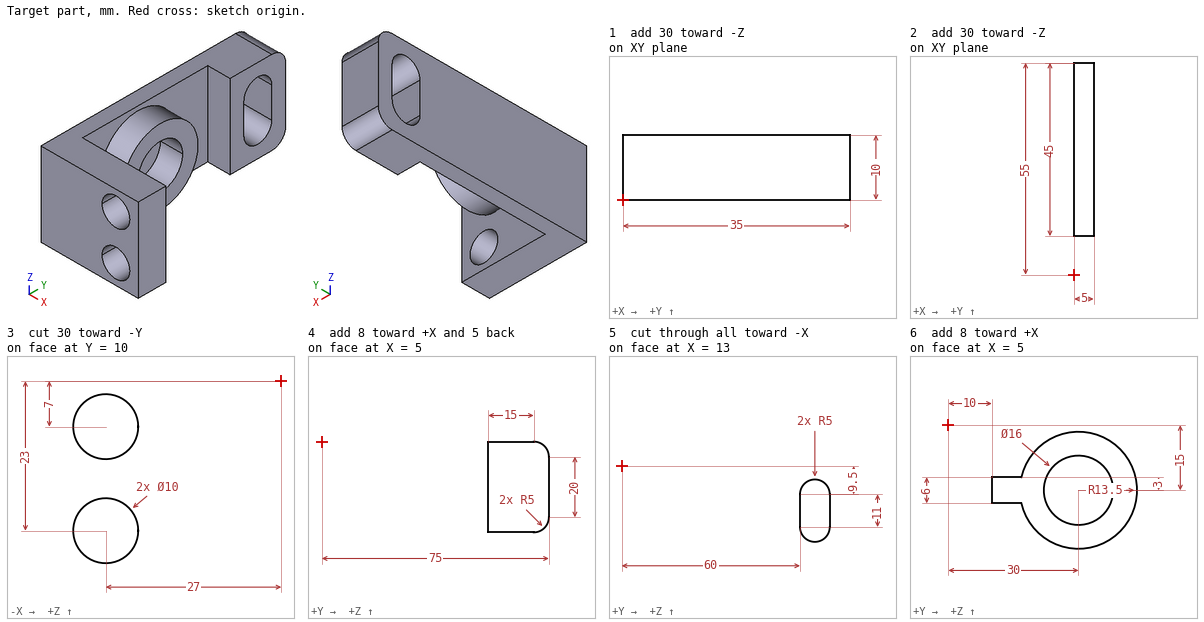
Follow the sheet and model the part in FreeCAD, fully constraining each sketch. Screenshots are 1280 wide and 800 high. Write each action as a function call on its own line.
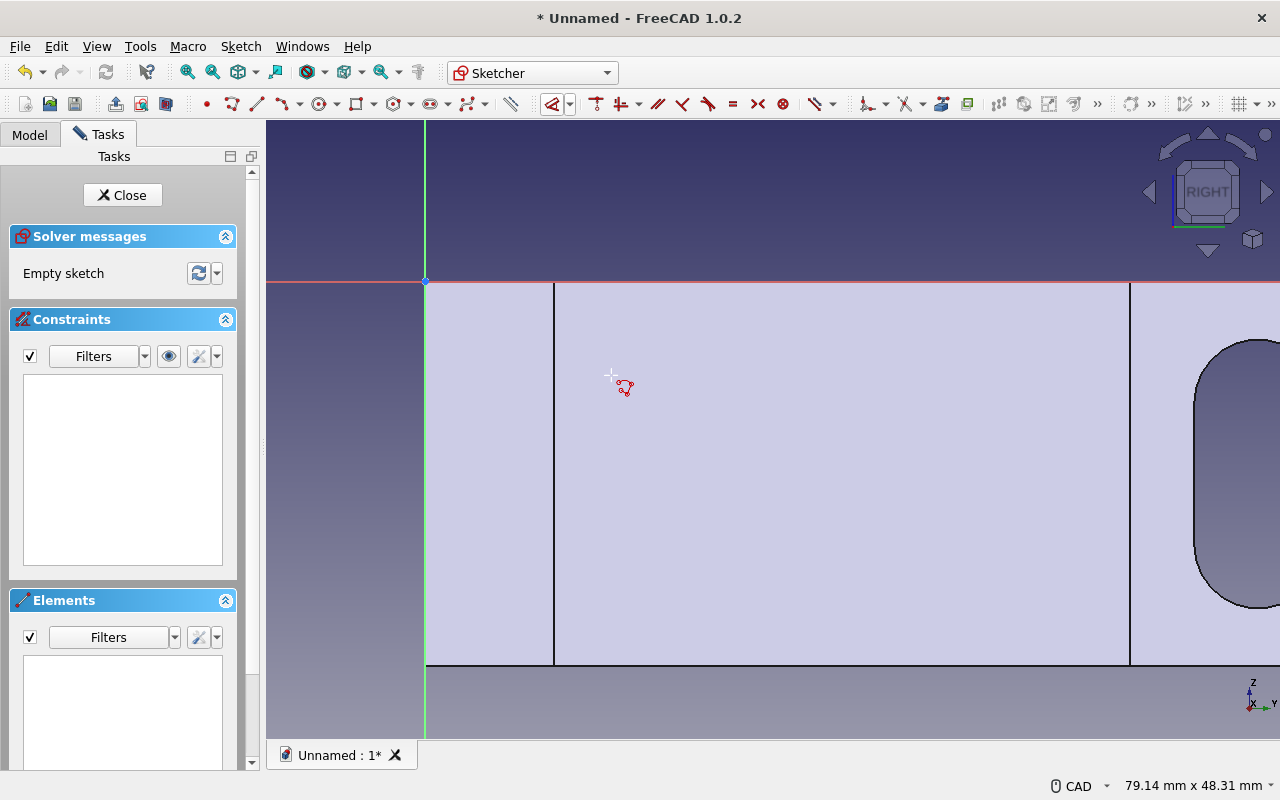
click(641, 436)
click(554, 436)
click(554, 512)
click(641, 512)
right_click(641, 512)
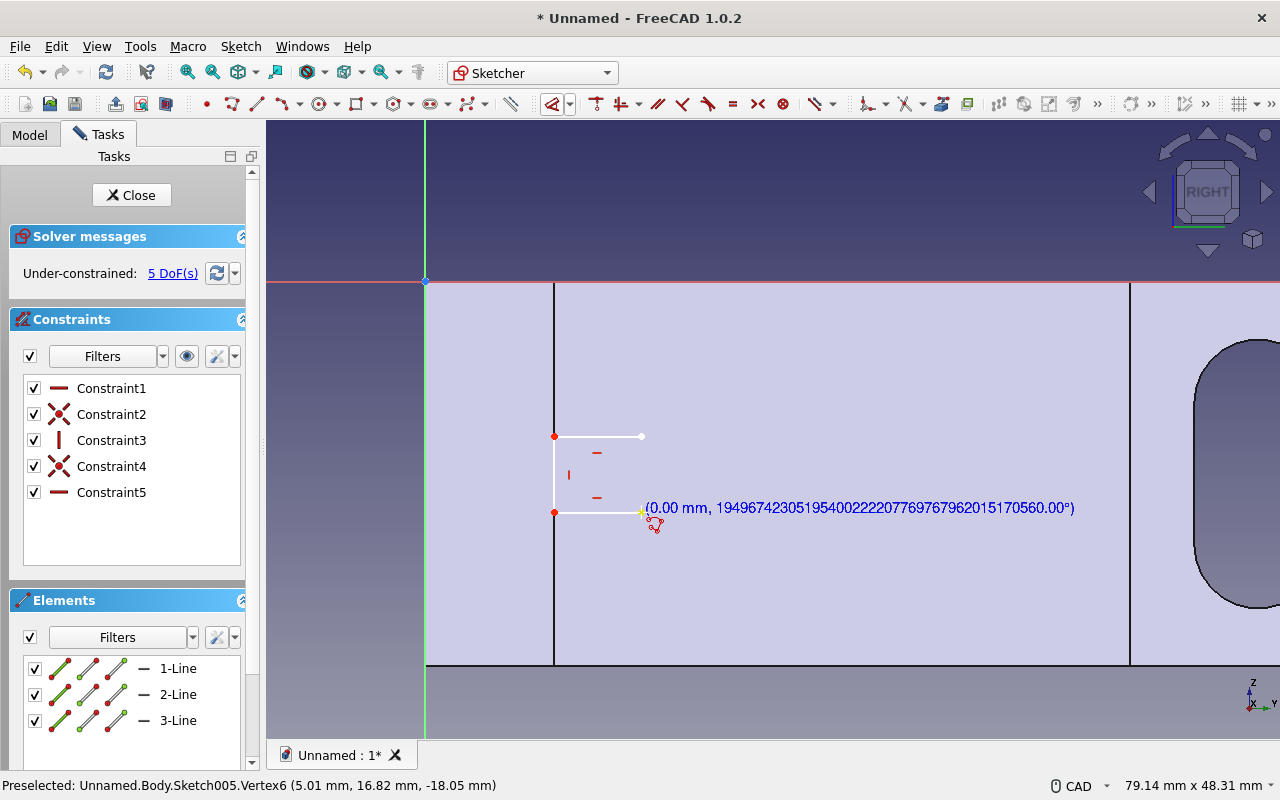
key(g)
key(3)
key(a)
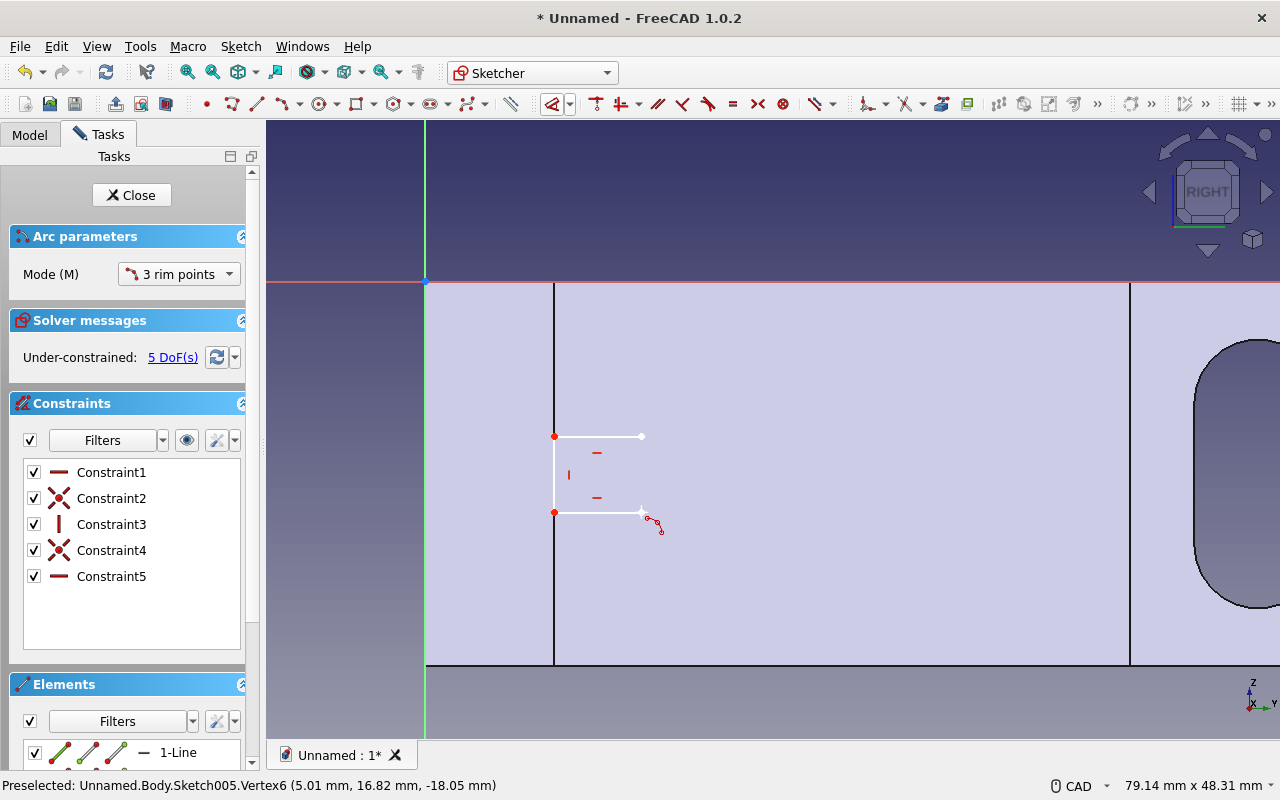
click(641, 513)
click(641, 437)
click(983, 474)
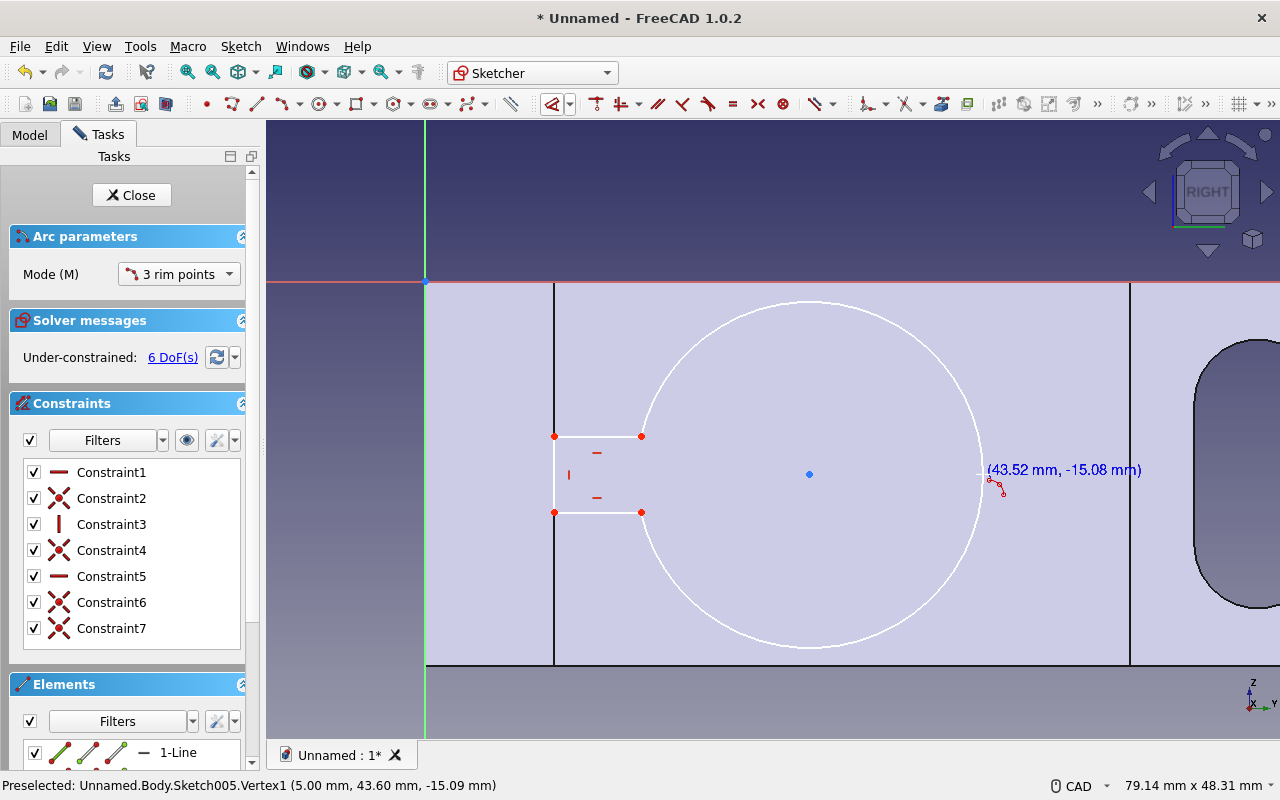
click(318, 104)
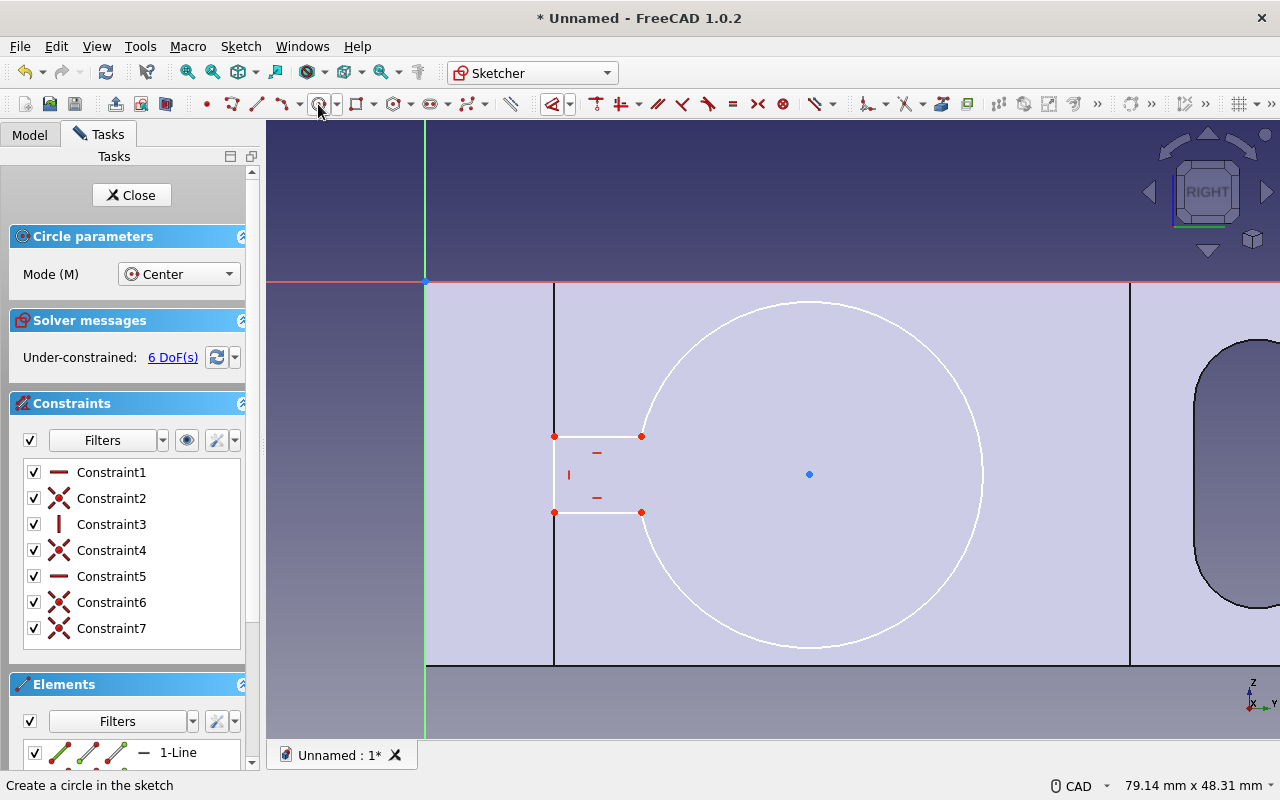
click(810, 474)
click(882, 401)
key(Escape)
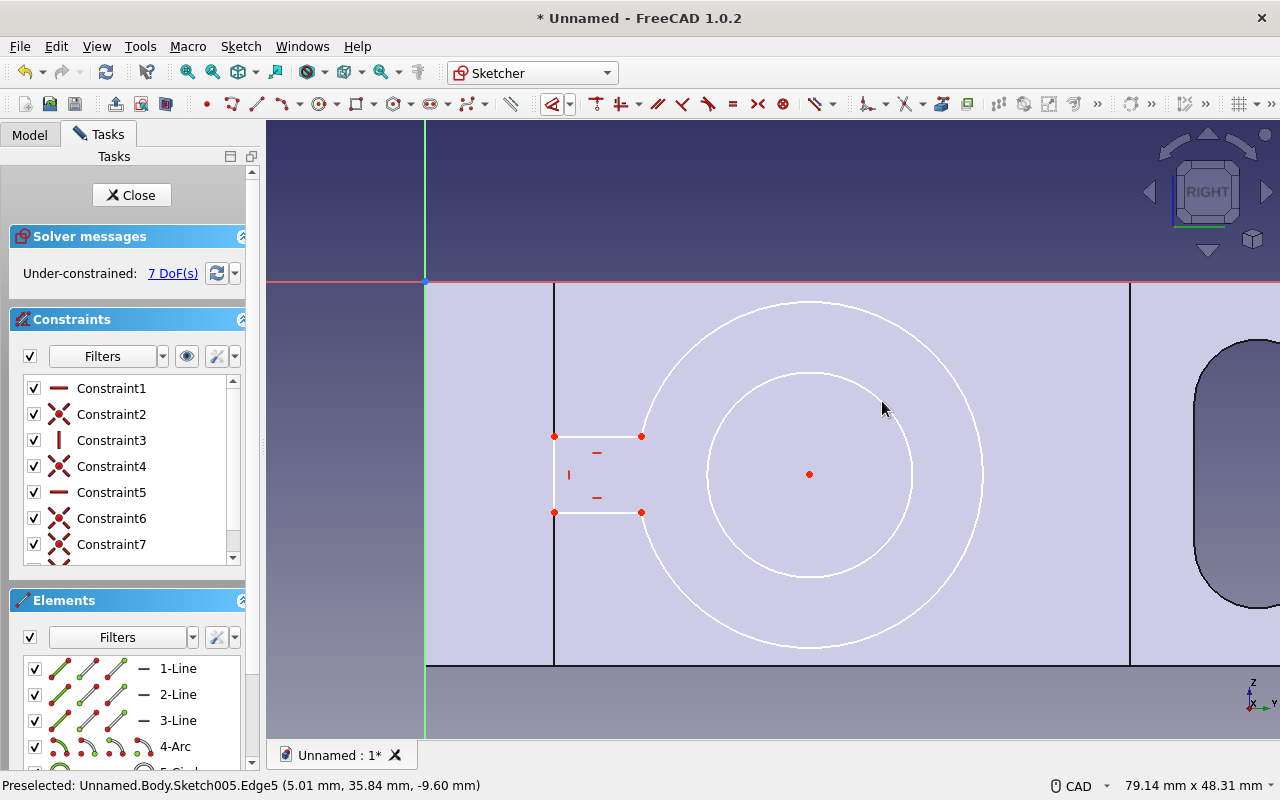
key(d)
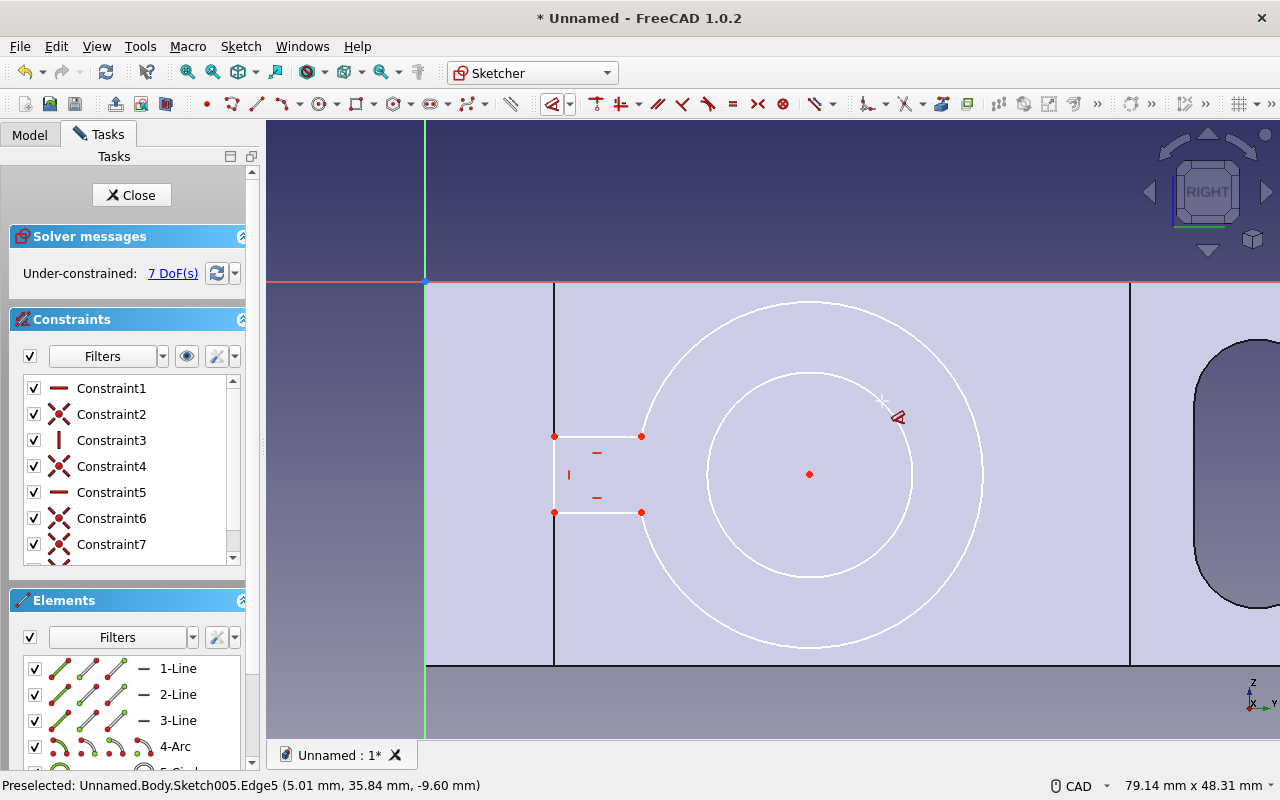
click(878, 634)
click(891, 663)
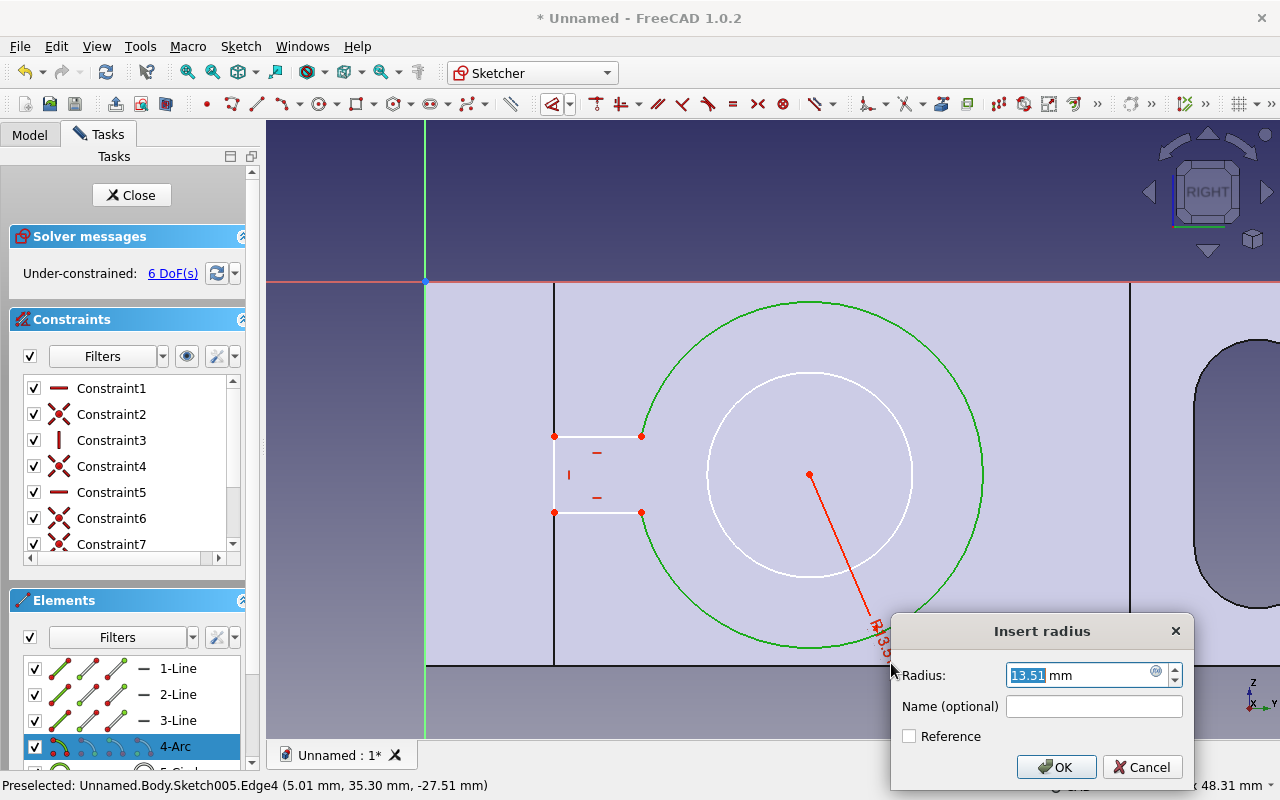
text(13.5)
key(Return)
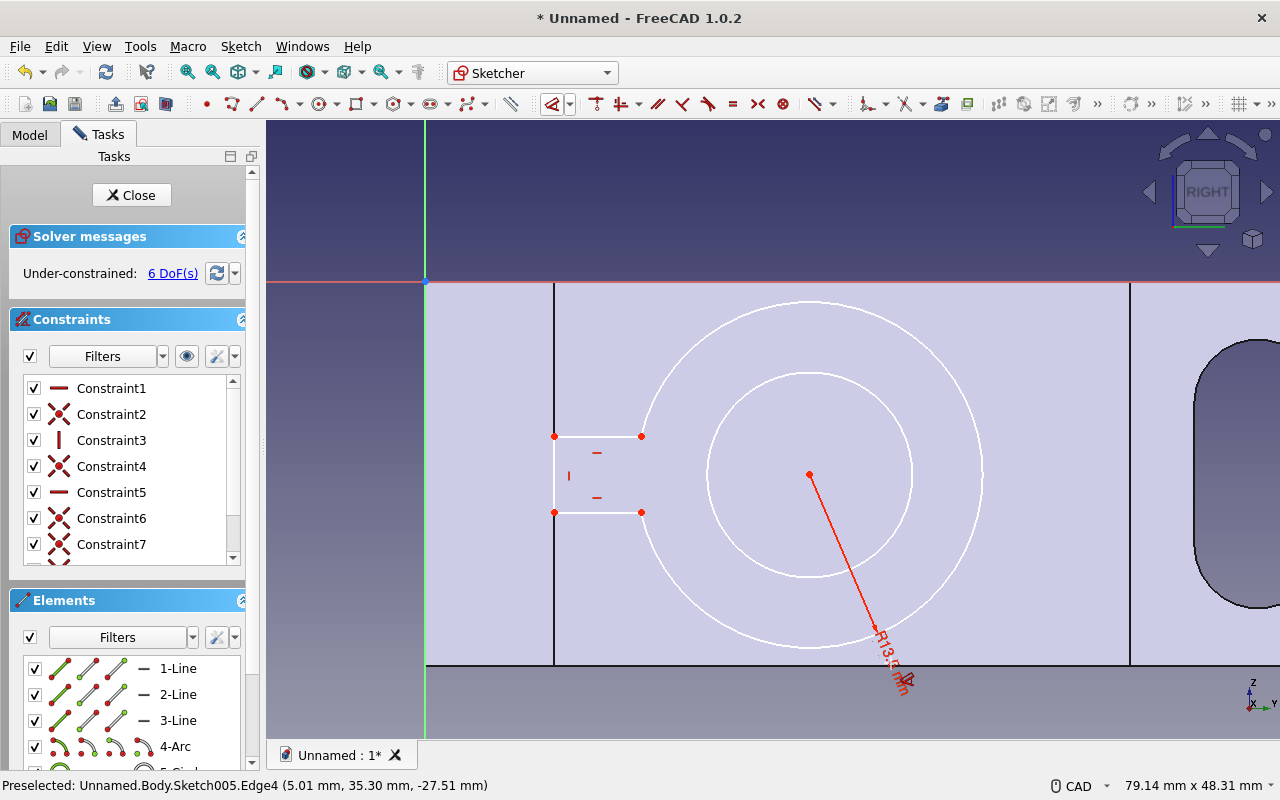
click(882, 402)
click(905, 379)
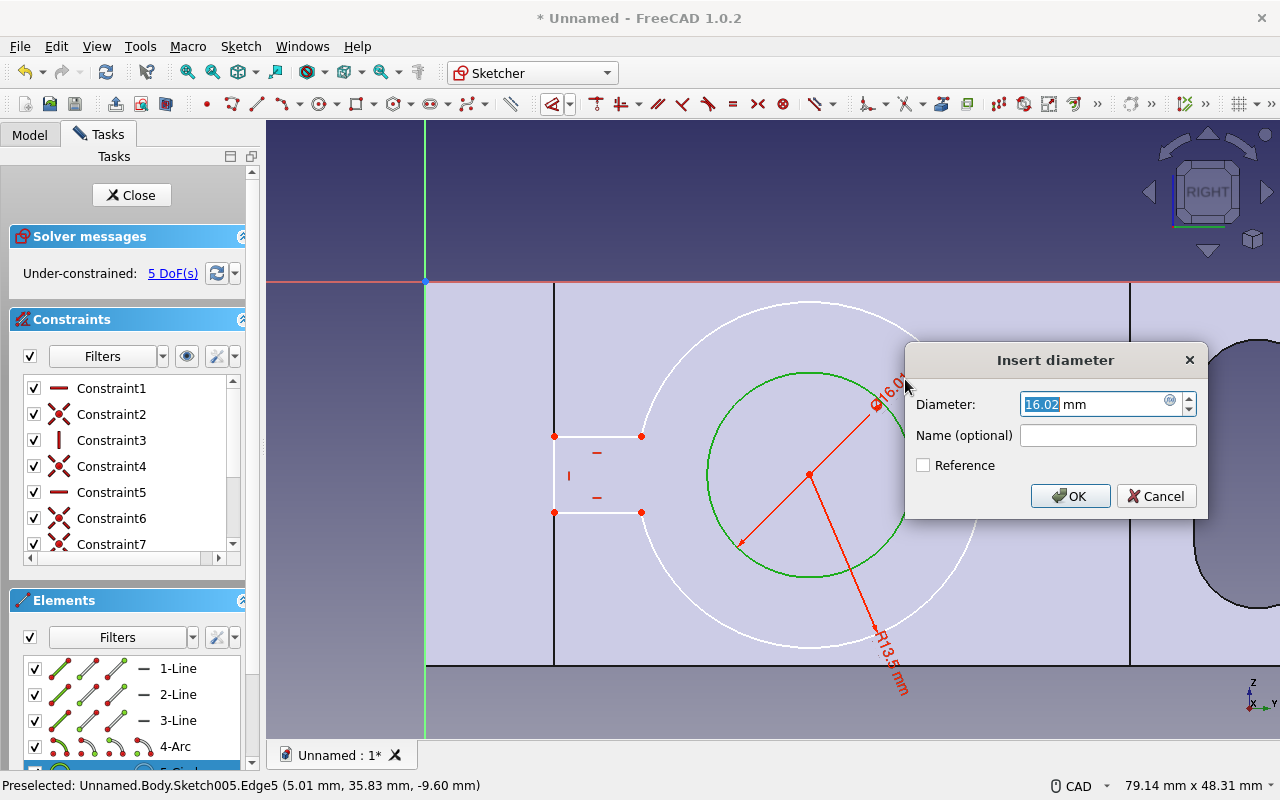
text(16)
key(Return)